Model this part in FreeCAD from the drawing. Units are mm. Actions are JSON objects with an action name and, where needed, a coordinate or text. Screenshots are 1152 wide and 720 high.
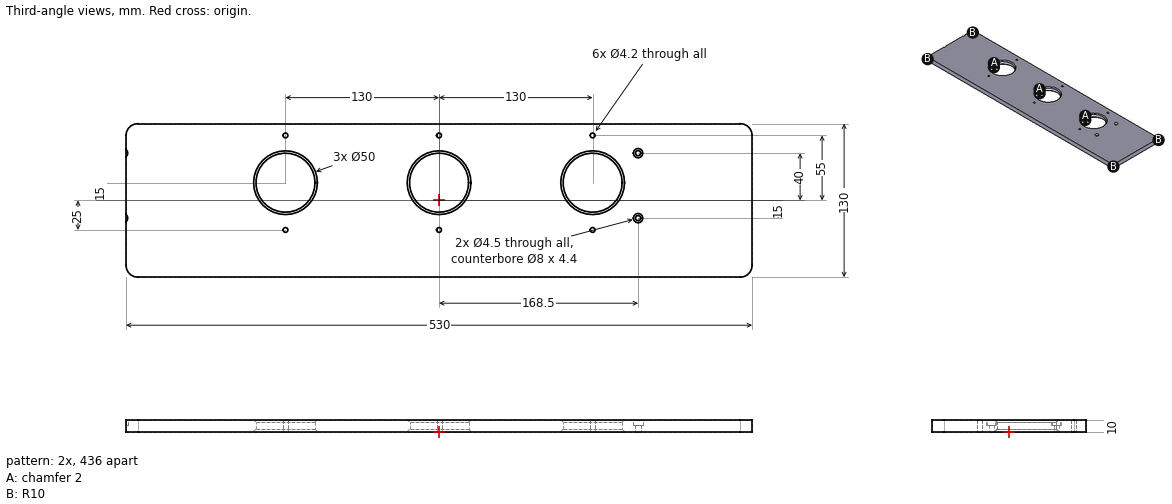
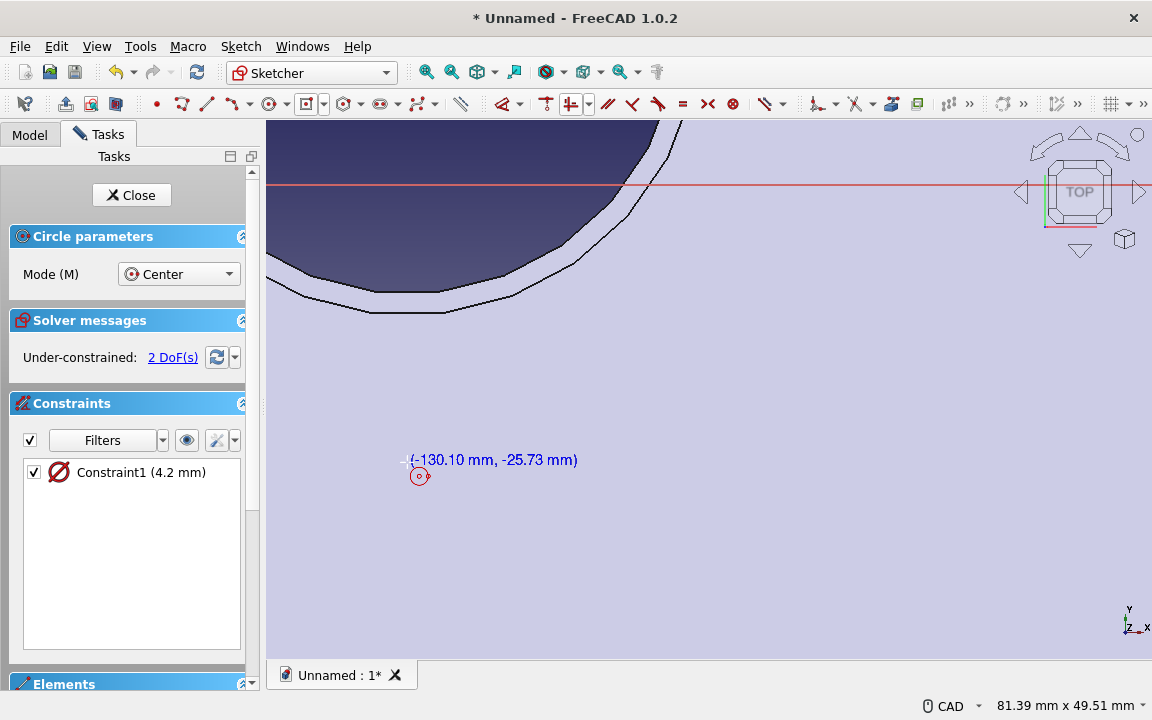
{"action": "scroll", "coordinate": [406, 462], "scroll_direction": "down", "scroll_amount": 9}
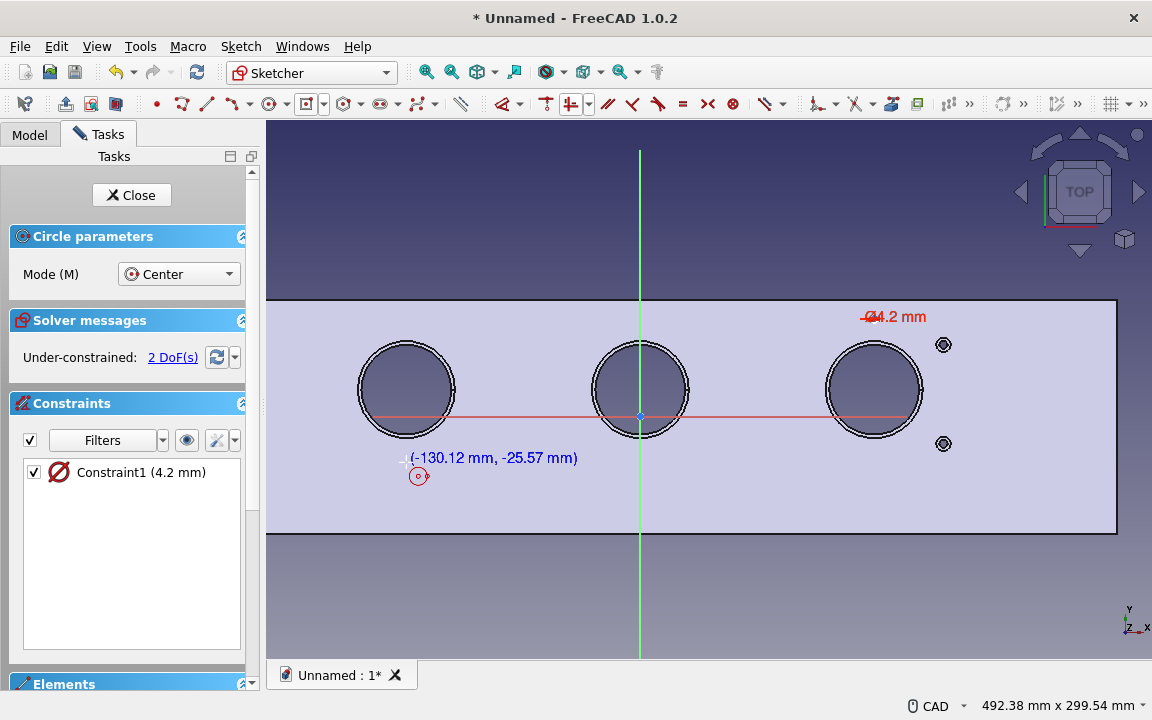
{"action": "left_click", "coordinate": [406, 462]}
{"action": "mouse_move", "coordinate": [409, 459]}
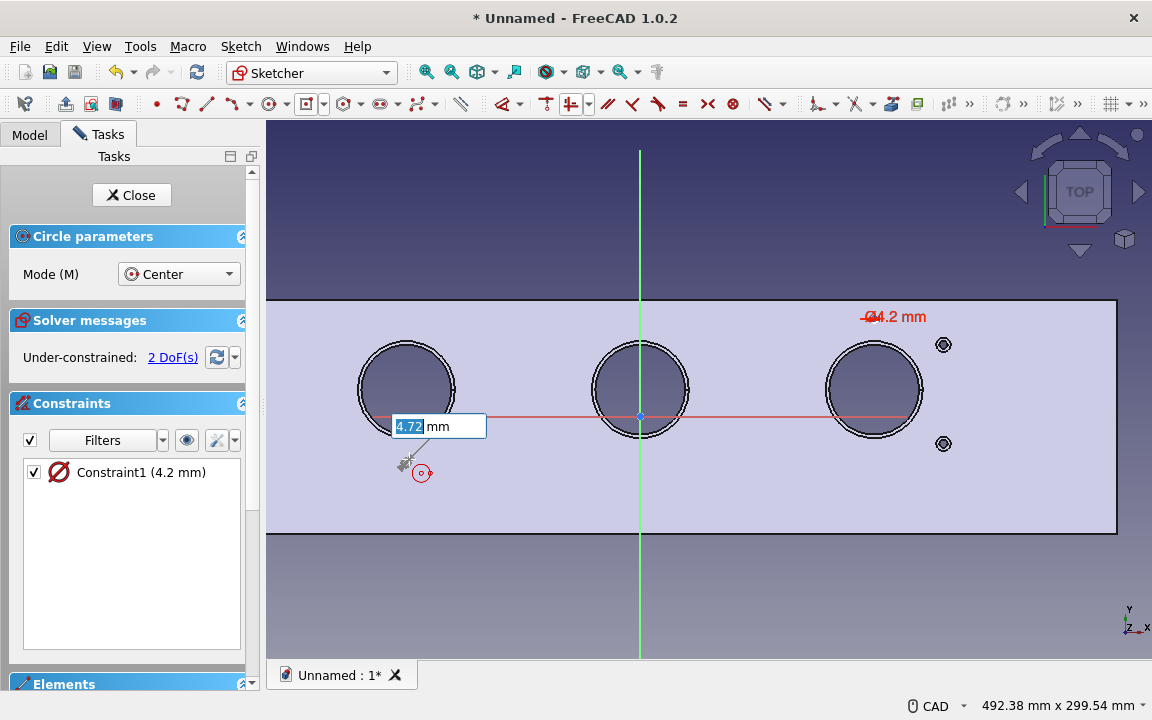
{"action": "type", "text": "4.2"}
{"action": "key", "text": "Return"}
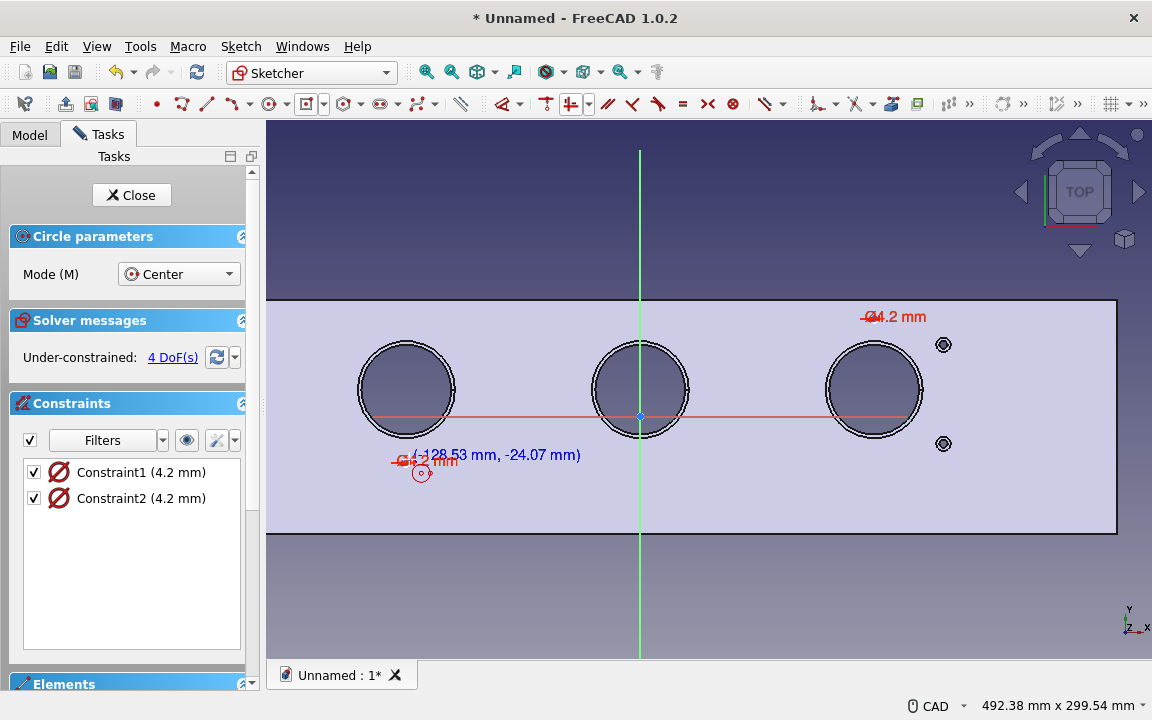
{"action": "scroll", "coordinate": [406, 318], "scroll_direction": "up", "scroll_amount": 9}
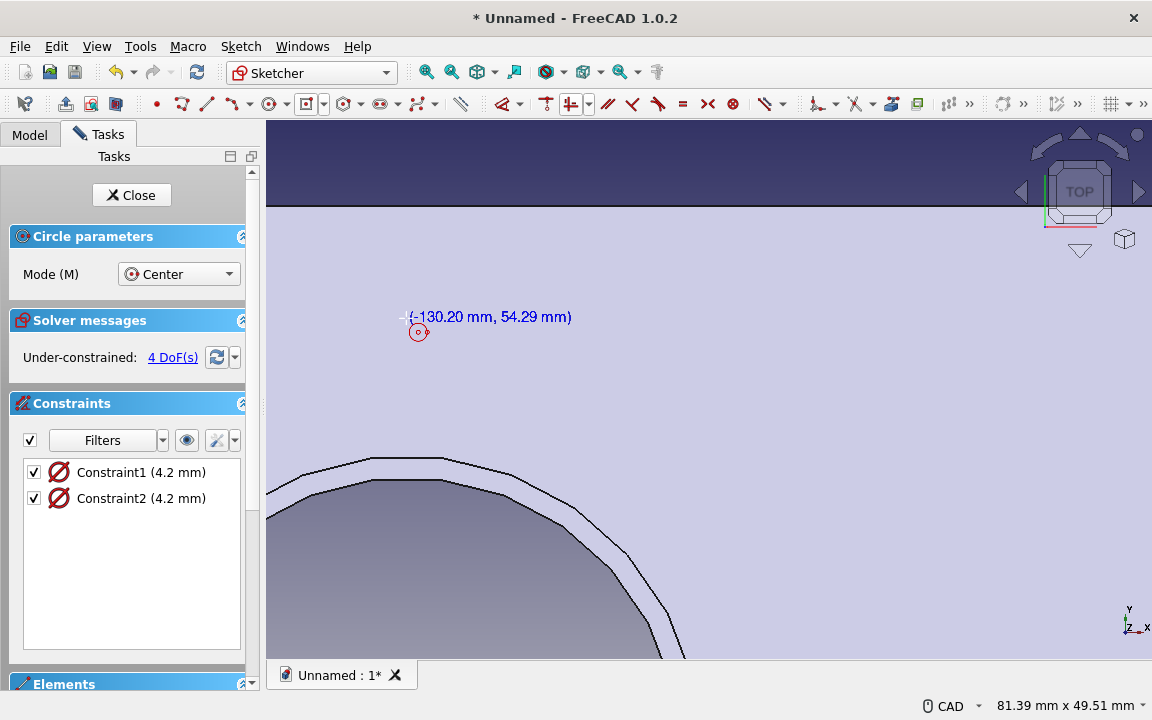
{"action": "scroll", "coordinate": [406, 318], "scroll_direction": "down", "scroll_amount": 9}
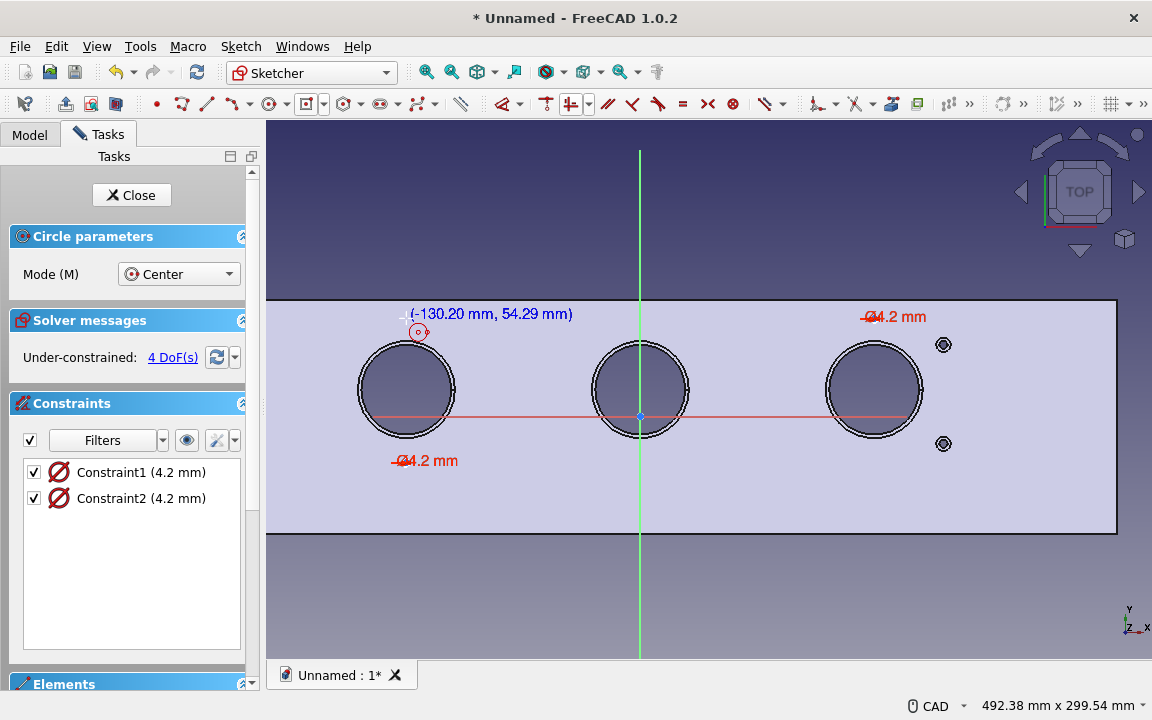
{"action": "left_click", "coordinate": [406, 318]}
{"action": "mouse_move", "coordinate": [409, 315]}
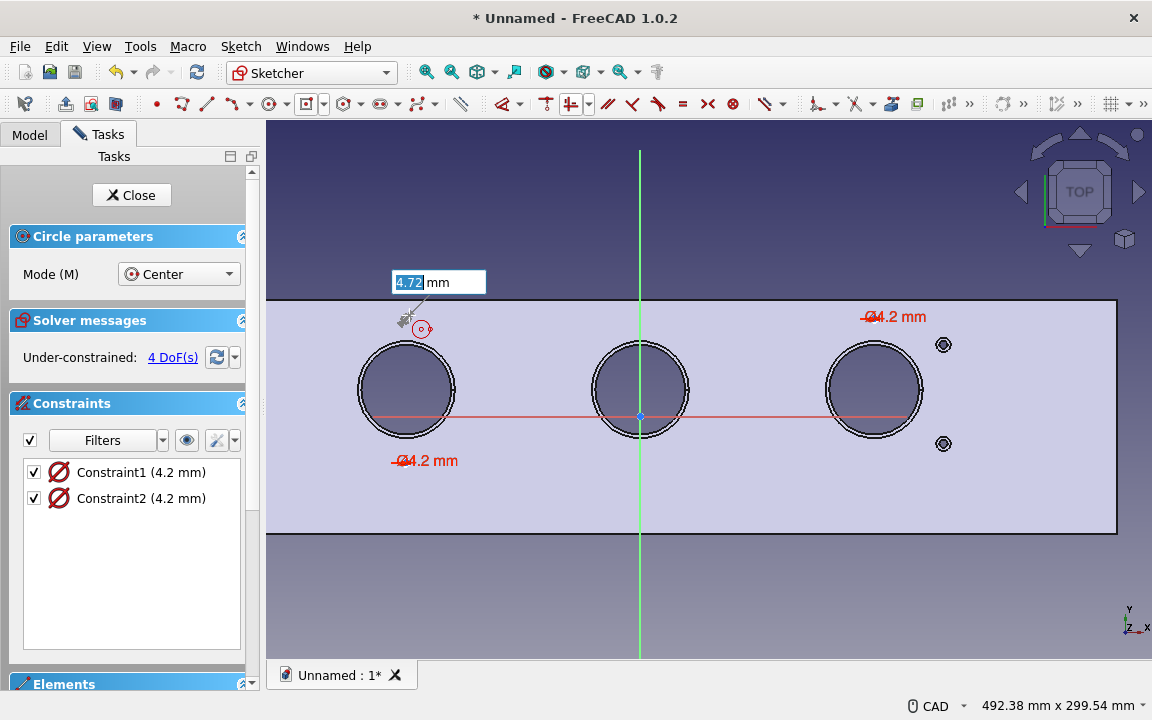
{"action": "type", "text": "4.2"}
{"action": "key", "text": "Return"}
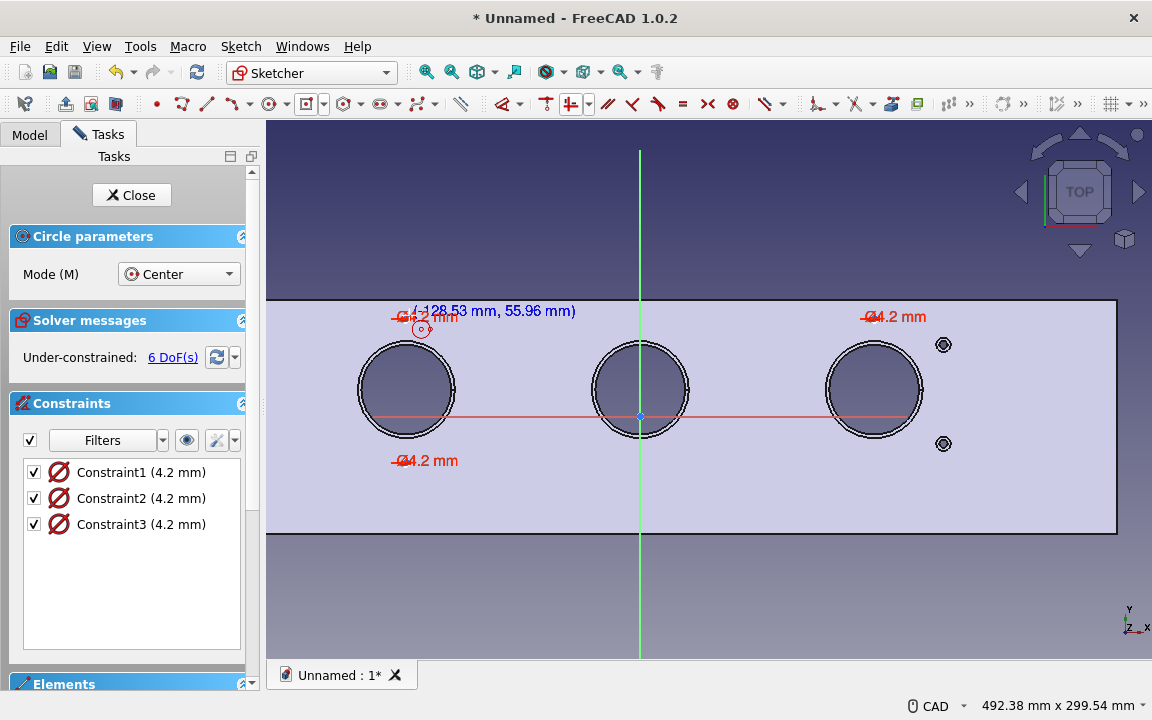
{"action": "scroll", "coordinate": [640, 318], "scroll_direction": "up", "scroll_amount": 9}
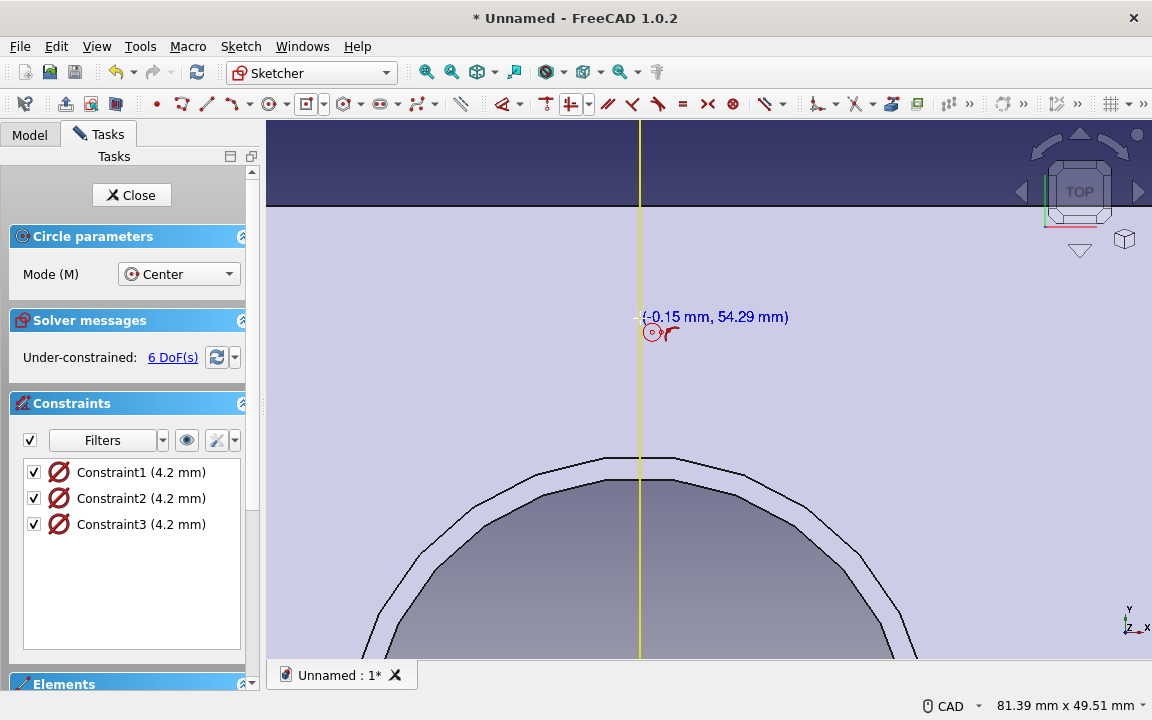
{"action": "scroll", "coordinate": [641, 318], "scroll_direction": "down", "scroll_amount": 9}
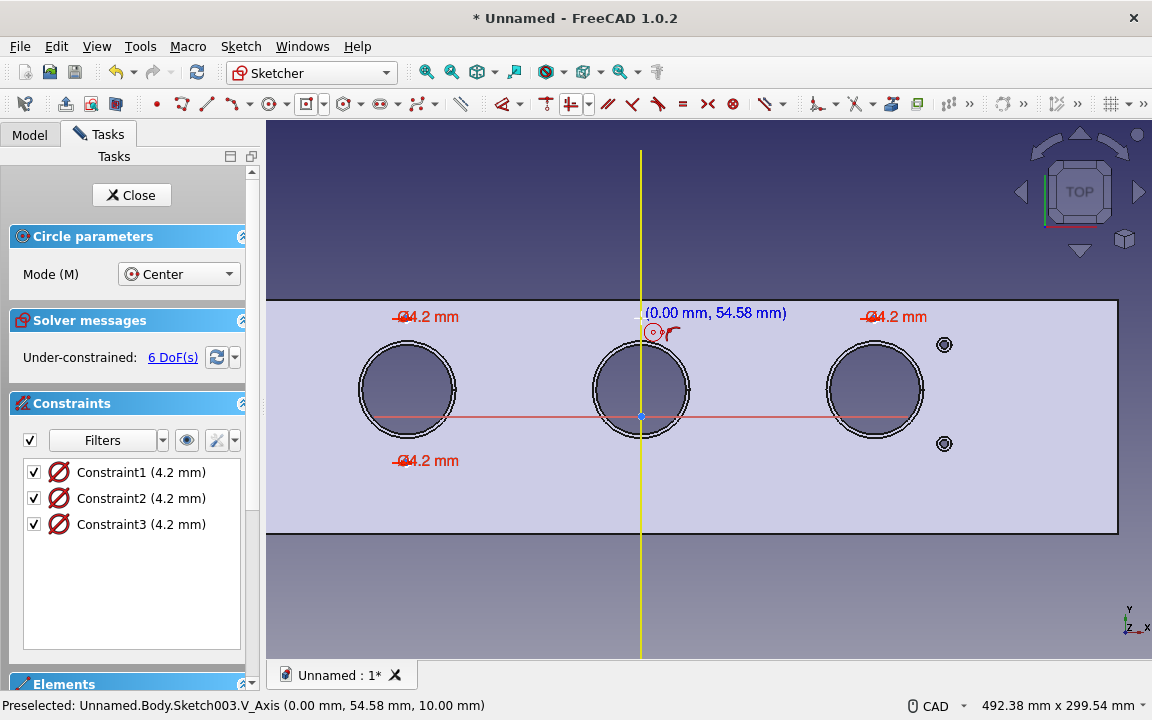
{"action": "left_click", "coordinate": [641, 318]}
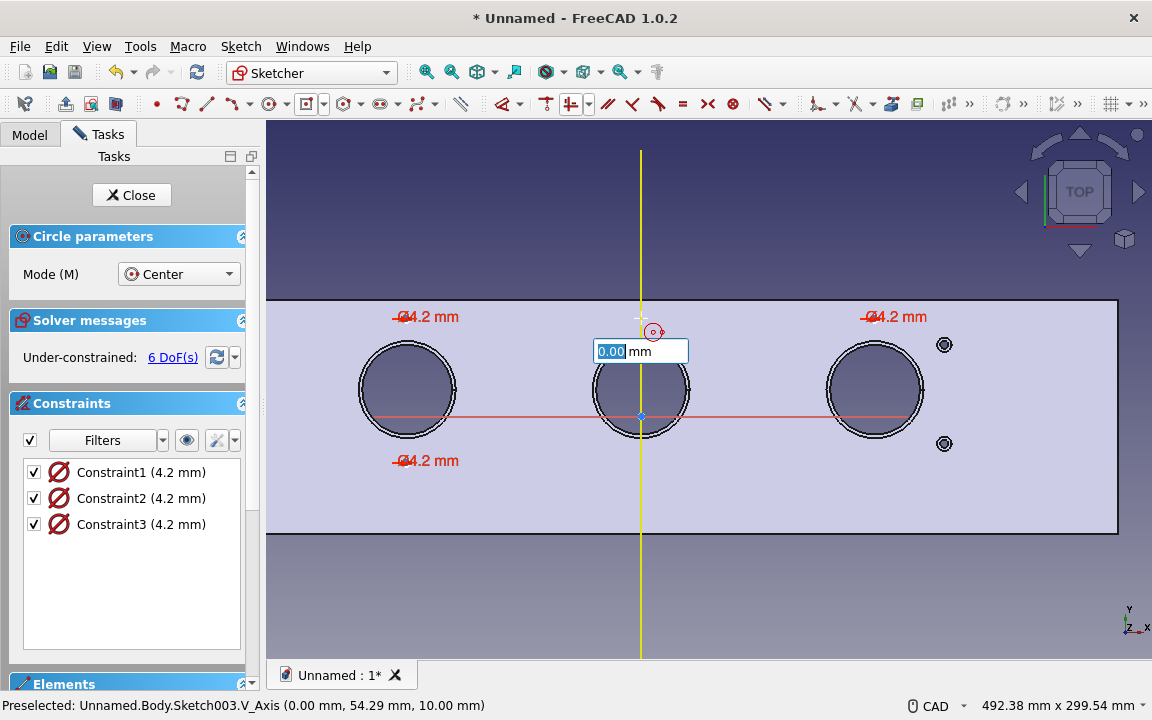
{"action": "scroll", "coordinate": [645, 316], "scroll_direction": "up", "scroll_amount": 8}
{"action": "mouse_move", "coordinate": [642, 317]}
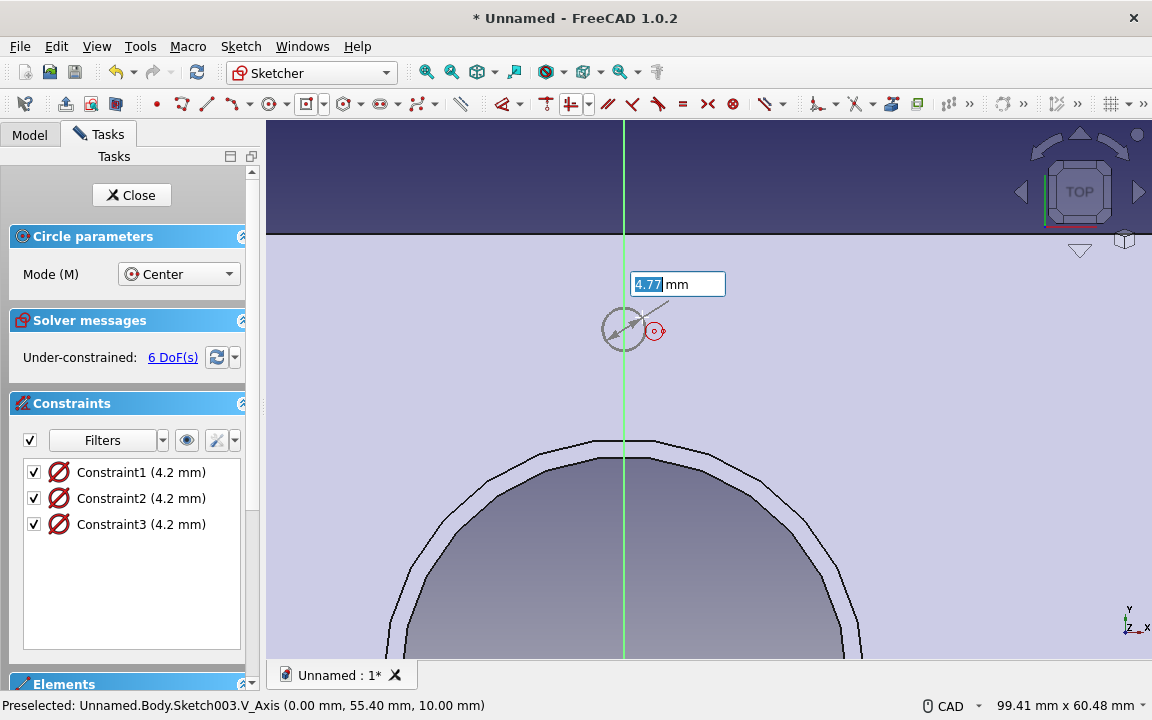
{"action": "type", "text": "4.2"}
{"action": "key", "text": "Return"}